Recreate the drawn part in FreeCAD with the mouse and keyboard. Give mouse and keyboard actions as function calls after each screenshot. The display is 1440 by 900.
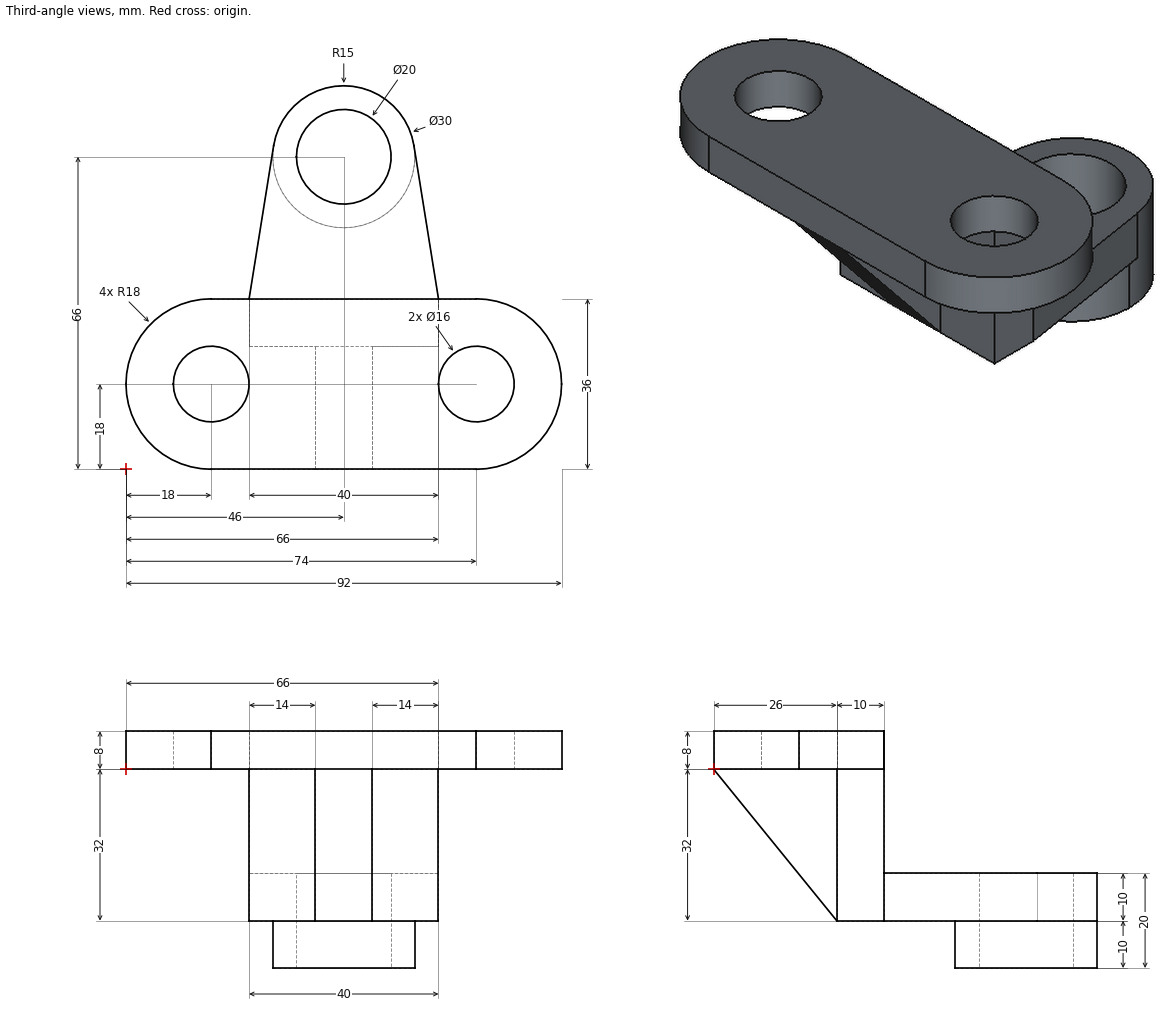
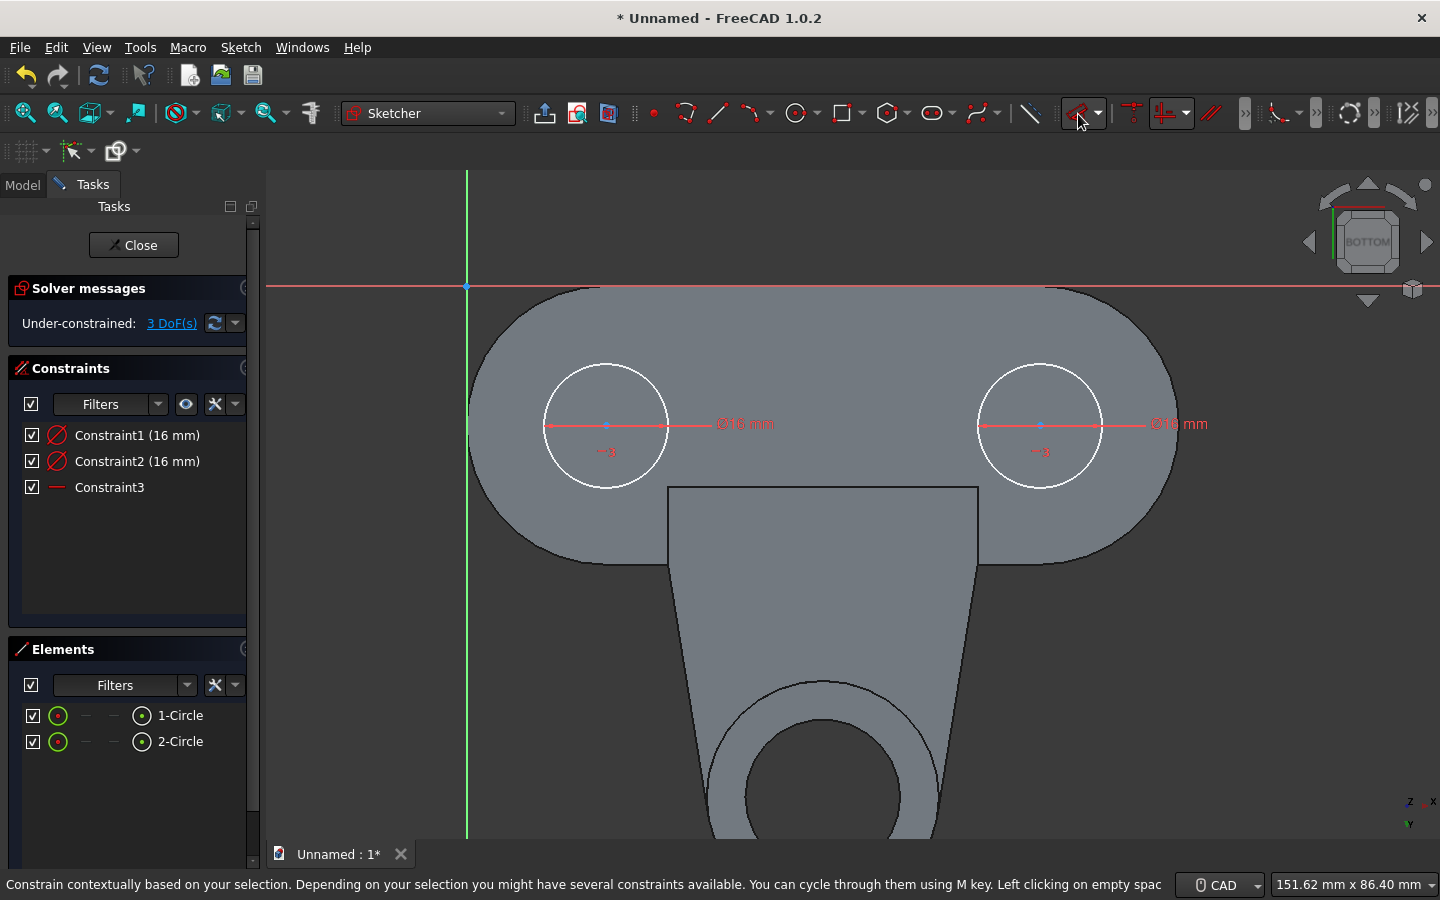
click(1040, 426)
click(753, 252)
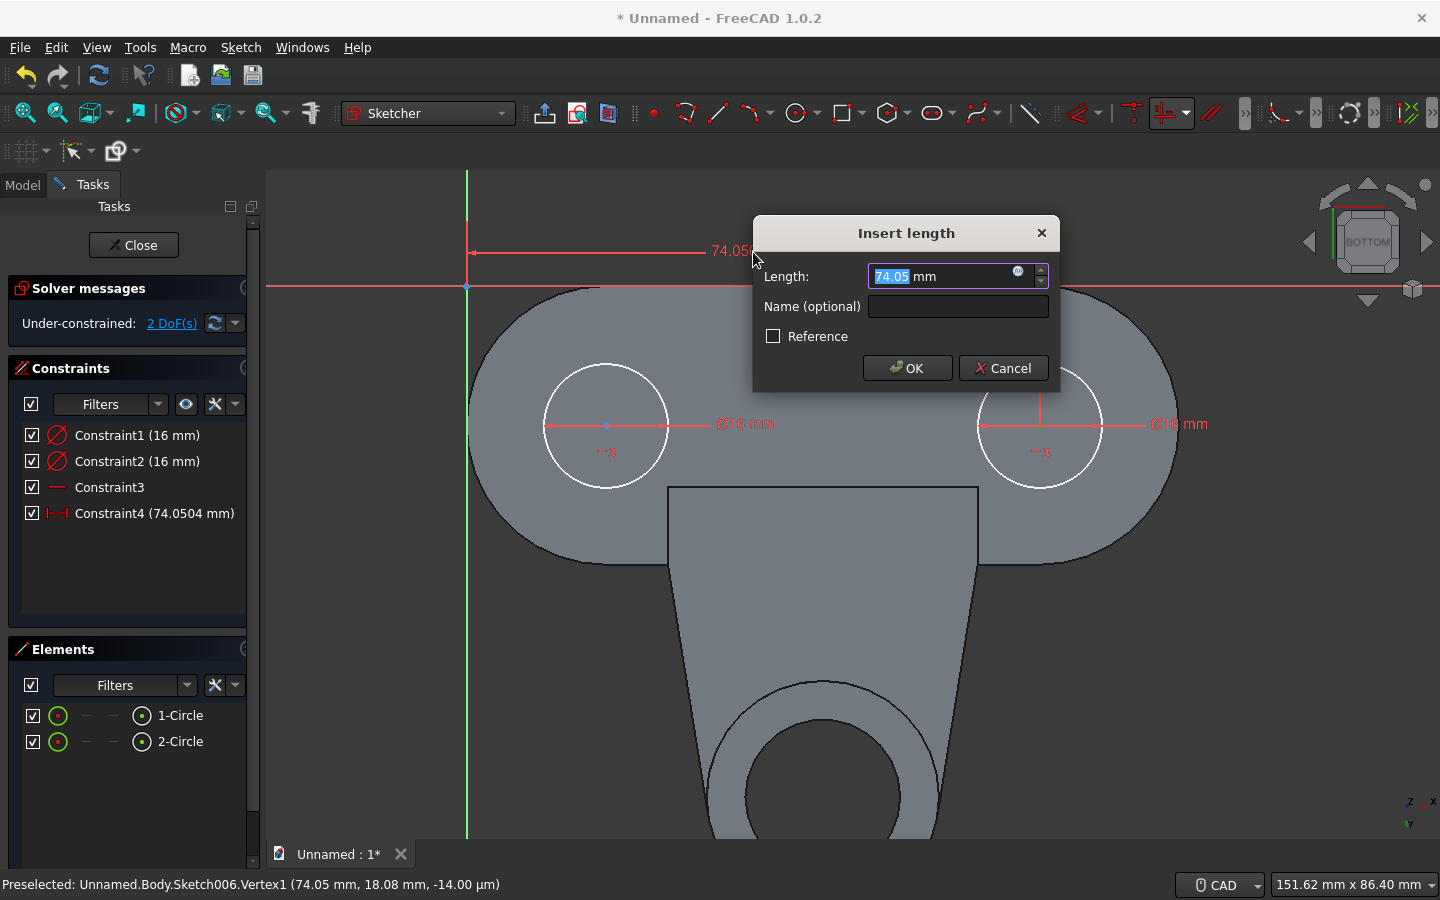
text(74)
key(Return)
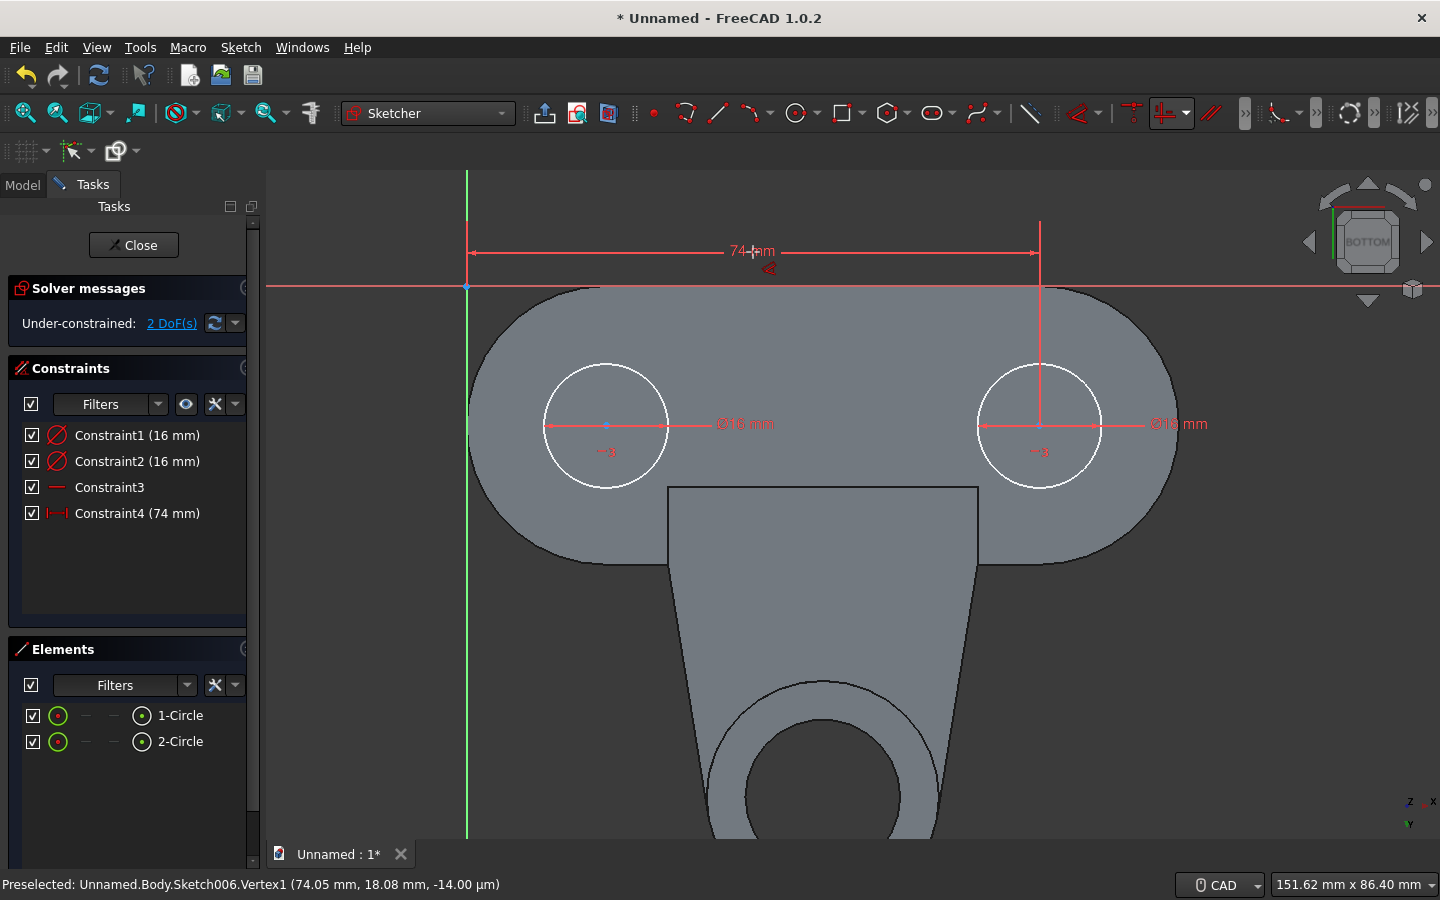
click(1040, 426)
click(433, 356)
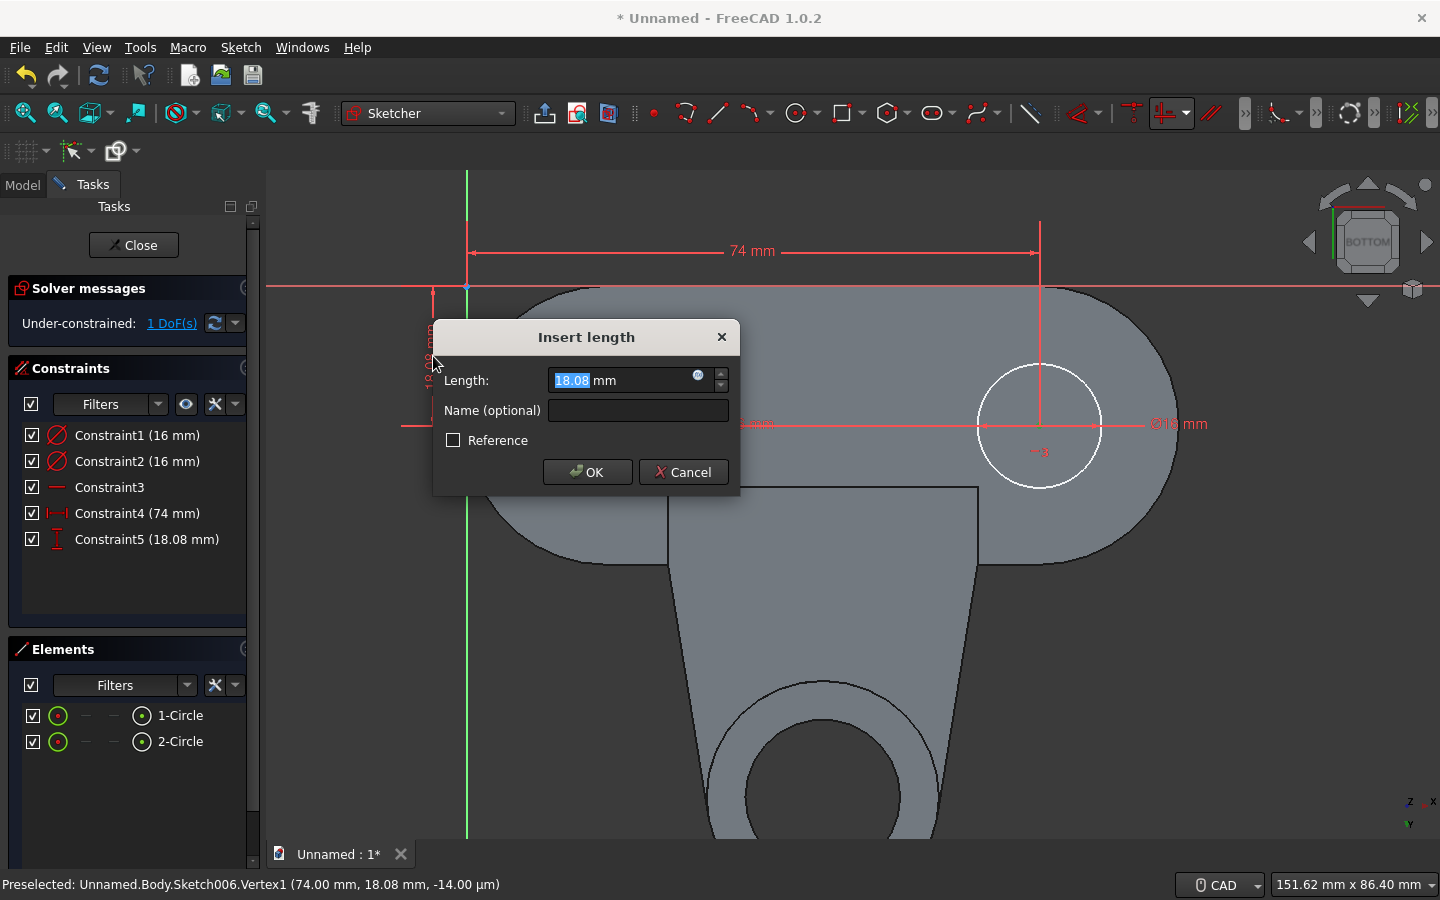
text(18)
key(Return)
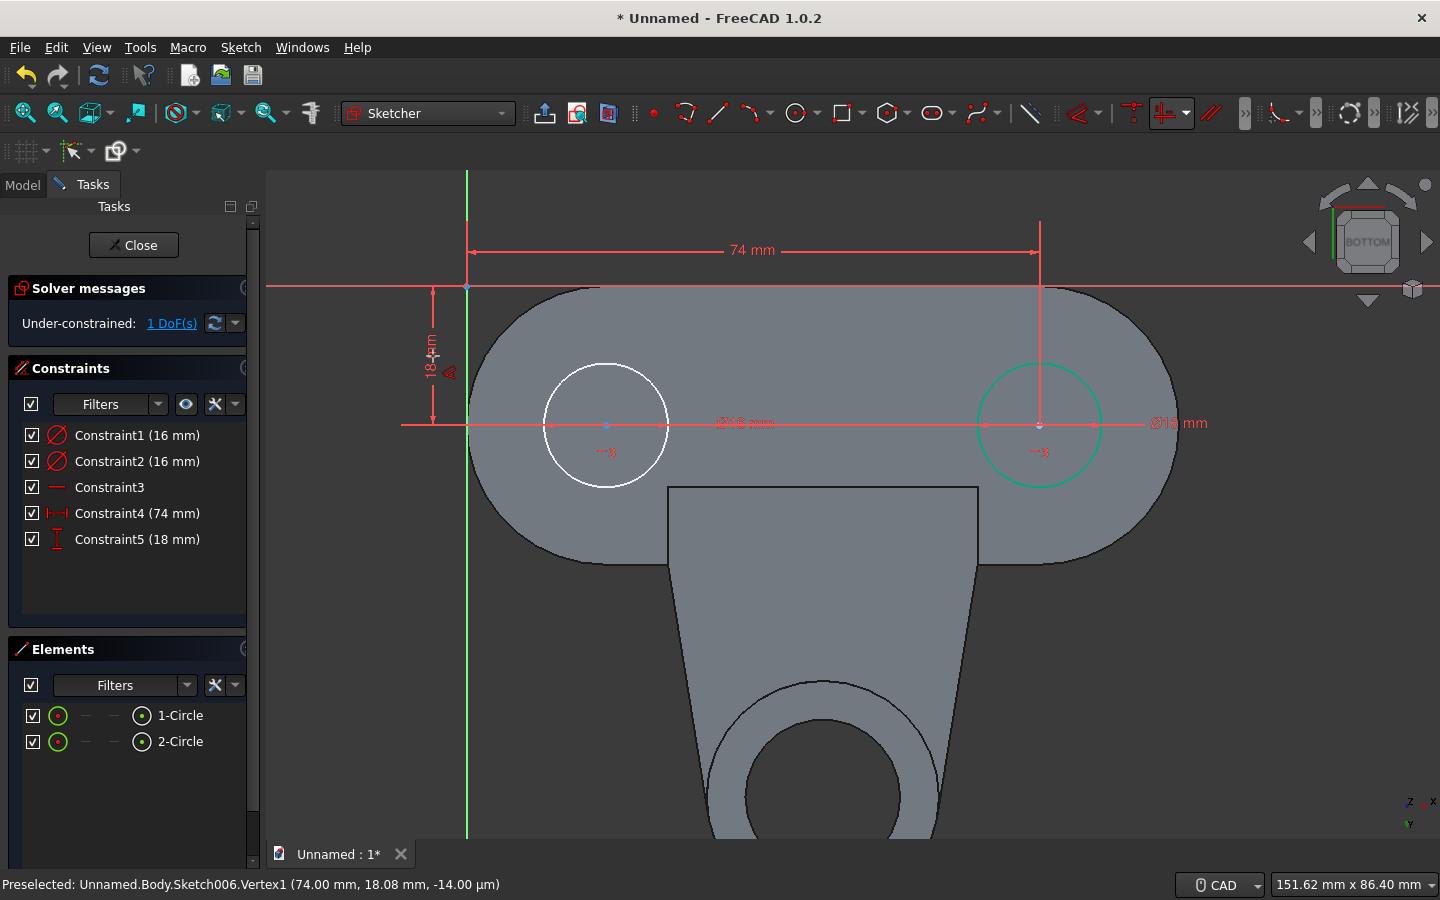
click(606, 425)
click(536, 252)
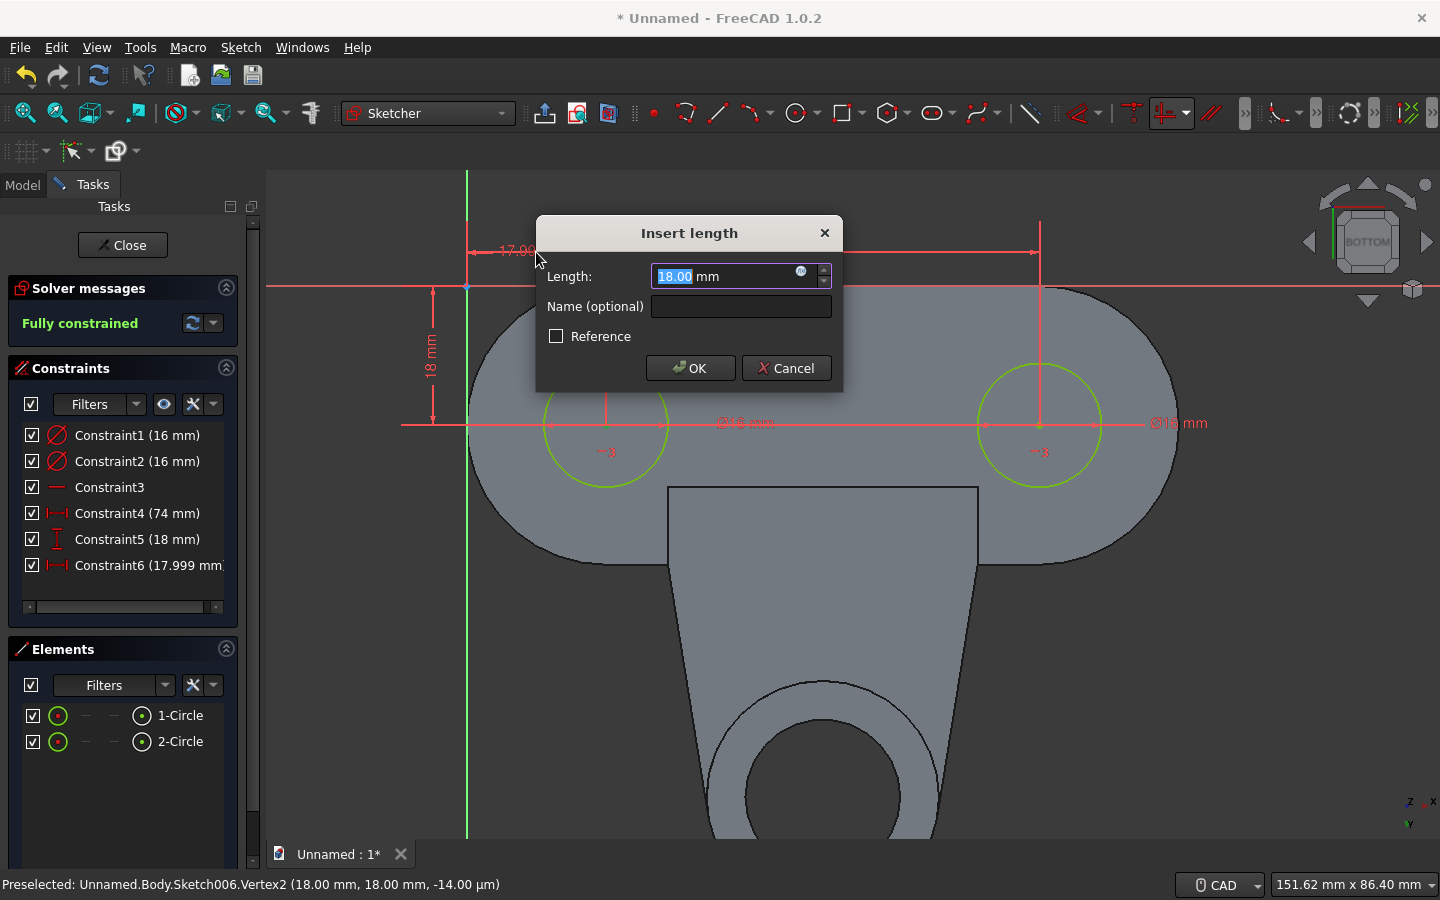
text(18)
key(Return)
key(Escape)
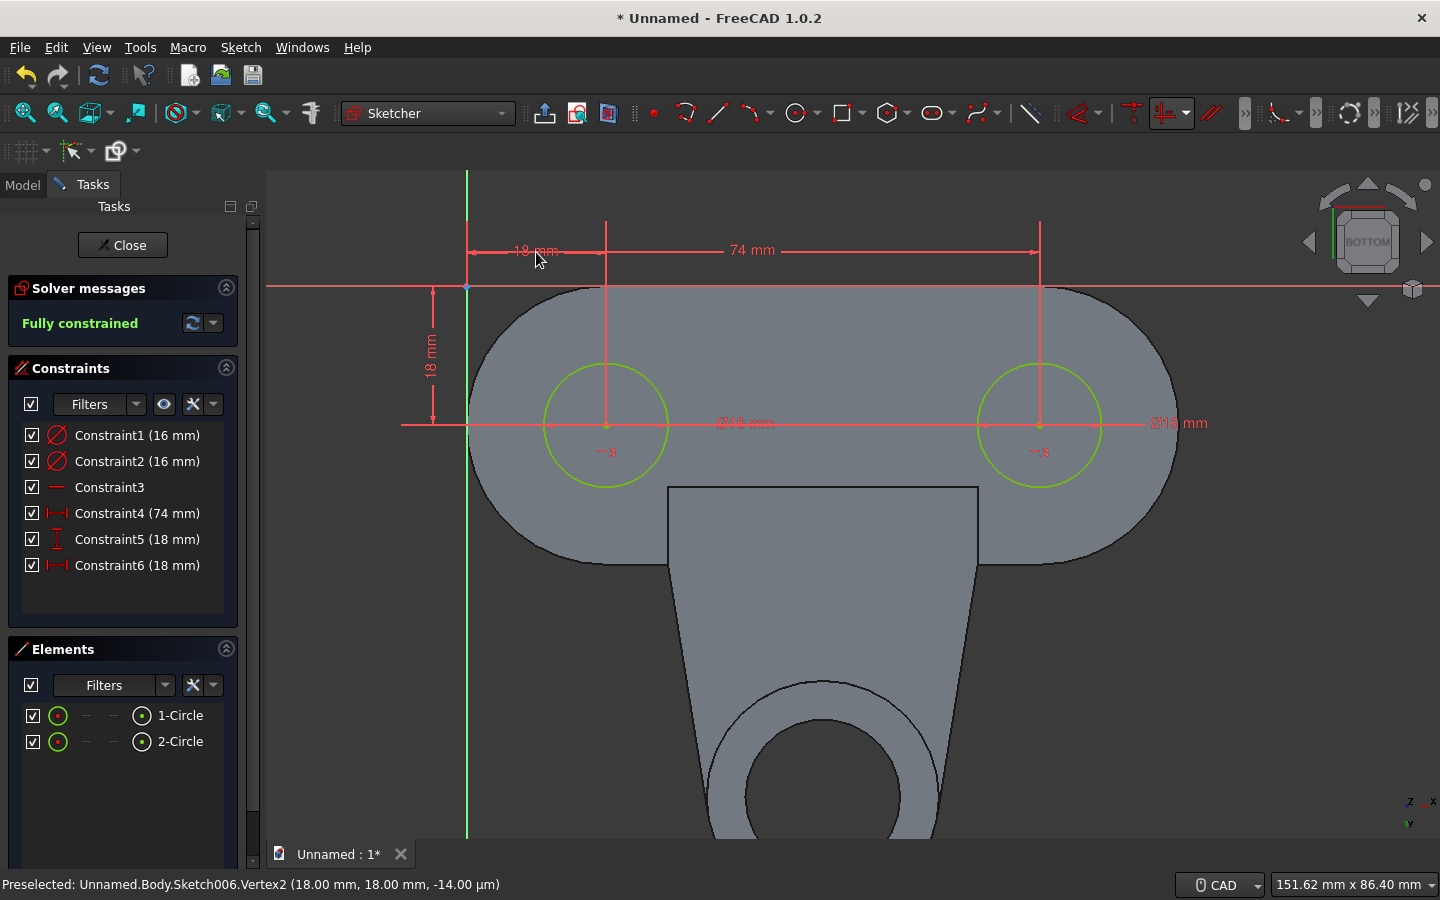
click(123, 245)